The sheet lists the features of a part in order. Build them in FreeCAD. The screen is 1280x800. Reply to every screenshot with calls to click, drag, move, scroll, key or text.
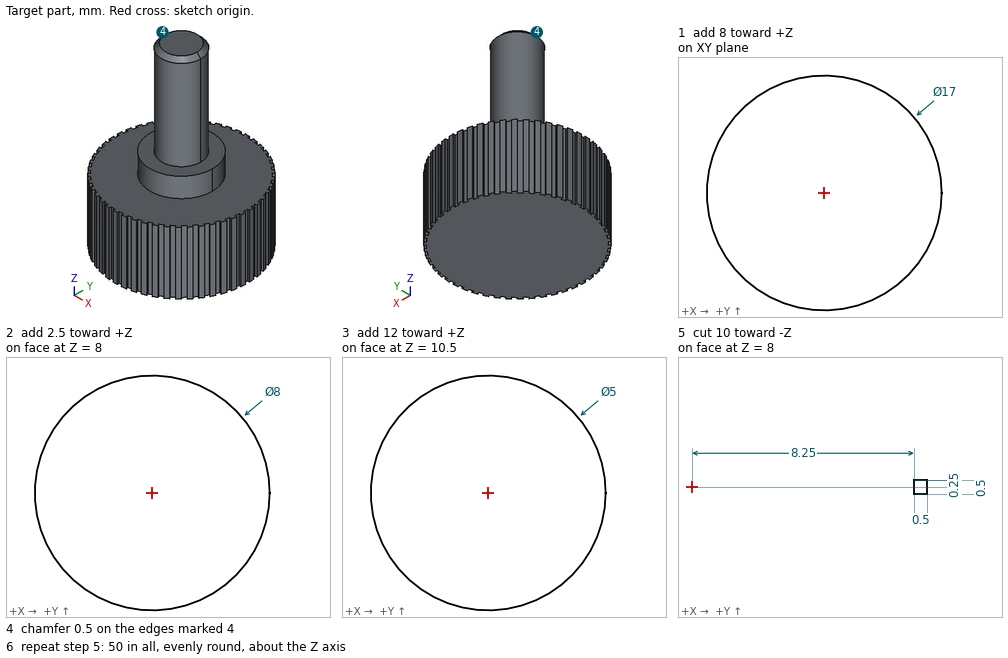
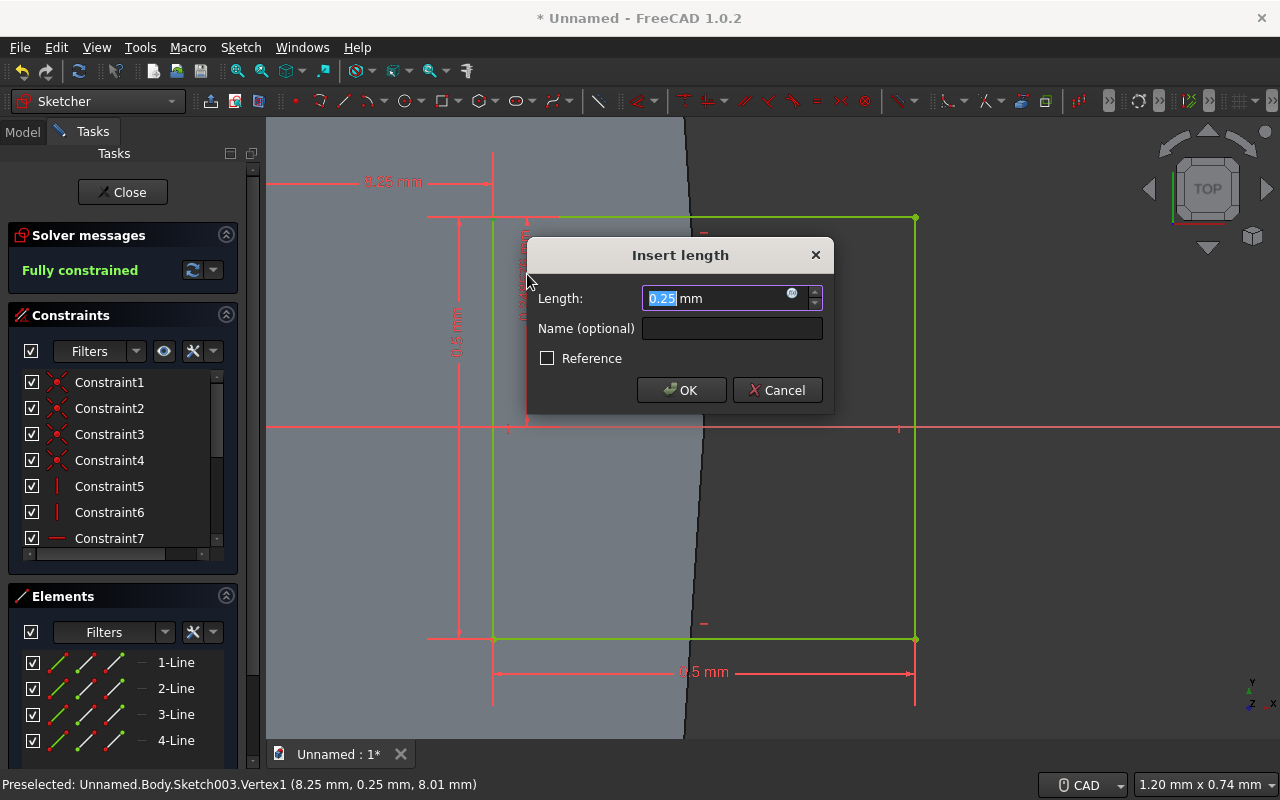
text(0.25)
key(Return)
key(Escape)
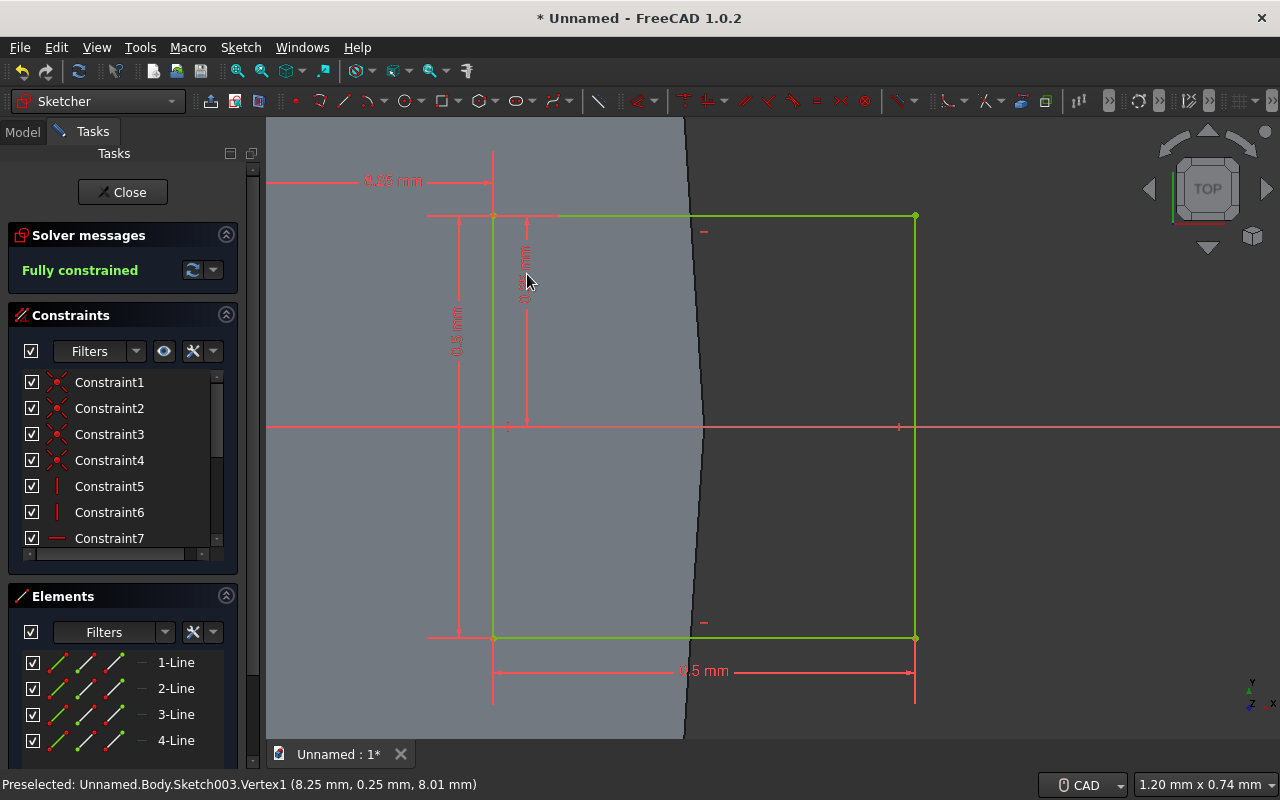
click(123, 192)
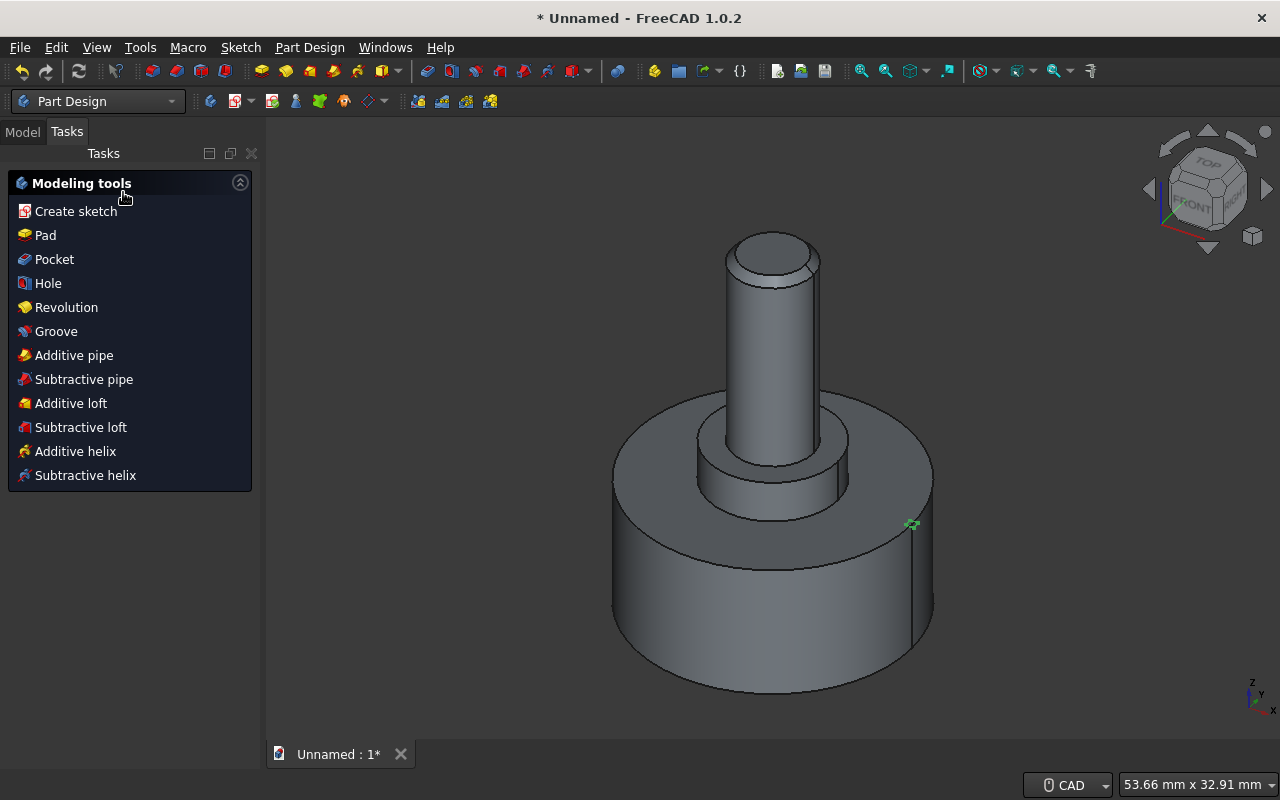
click(428, 72)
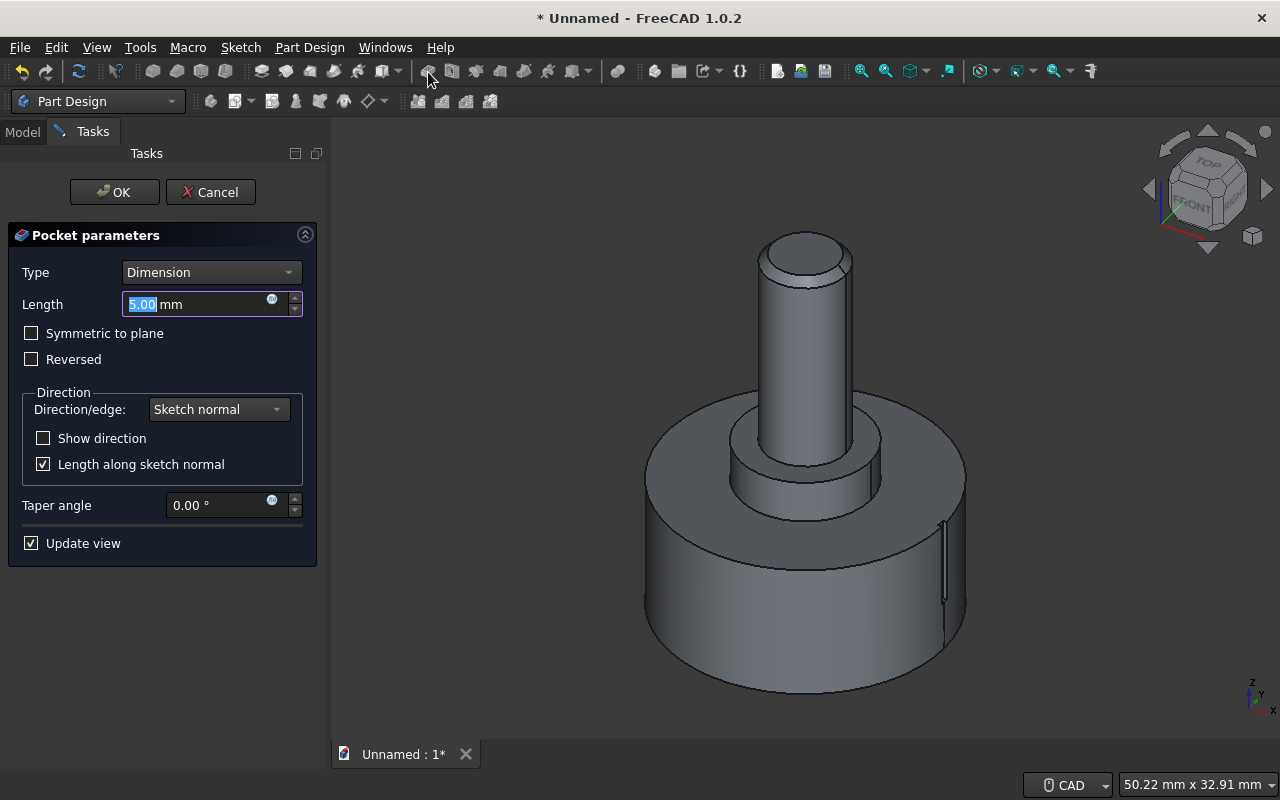
text(10)
key(Tab)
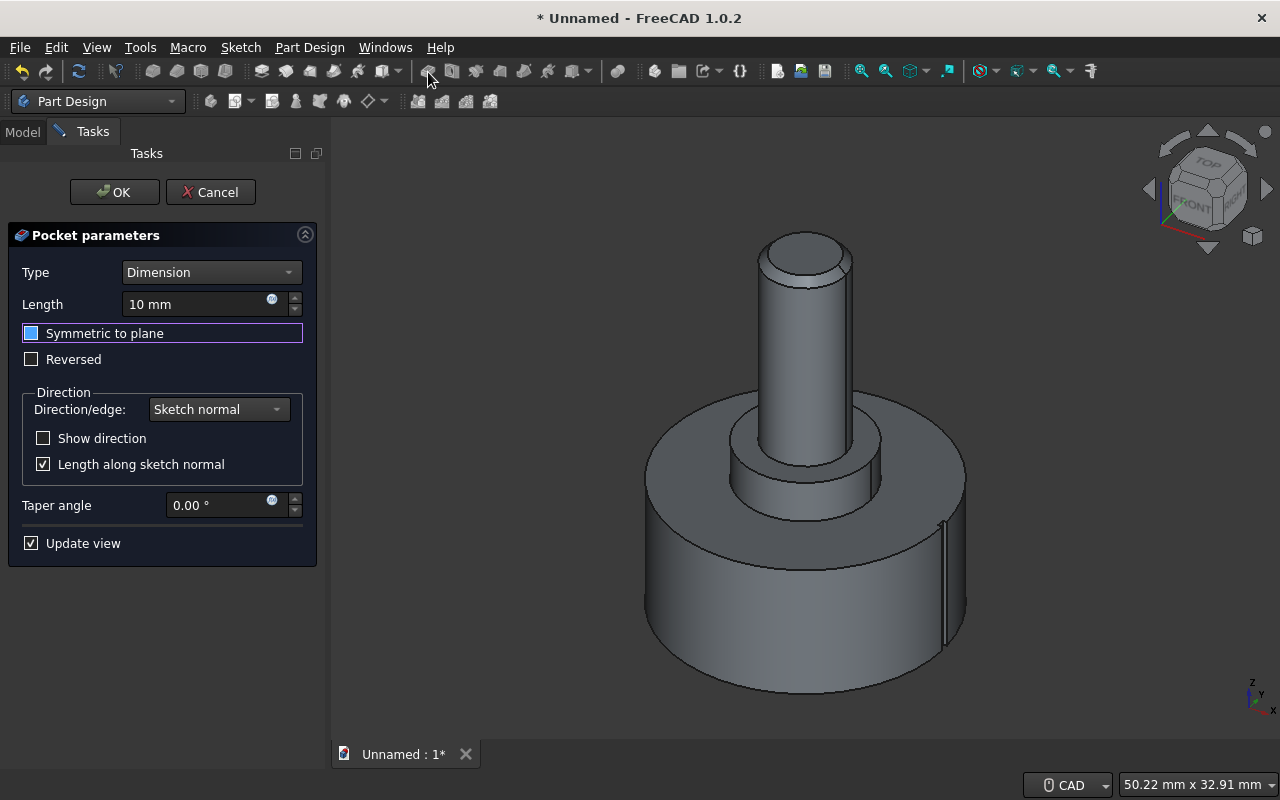
click(115, 192)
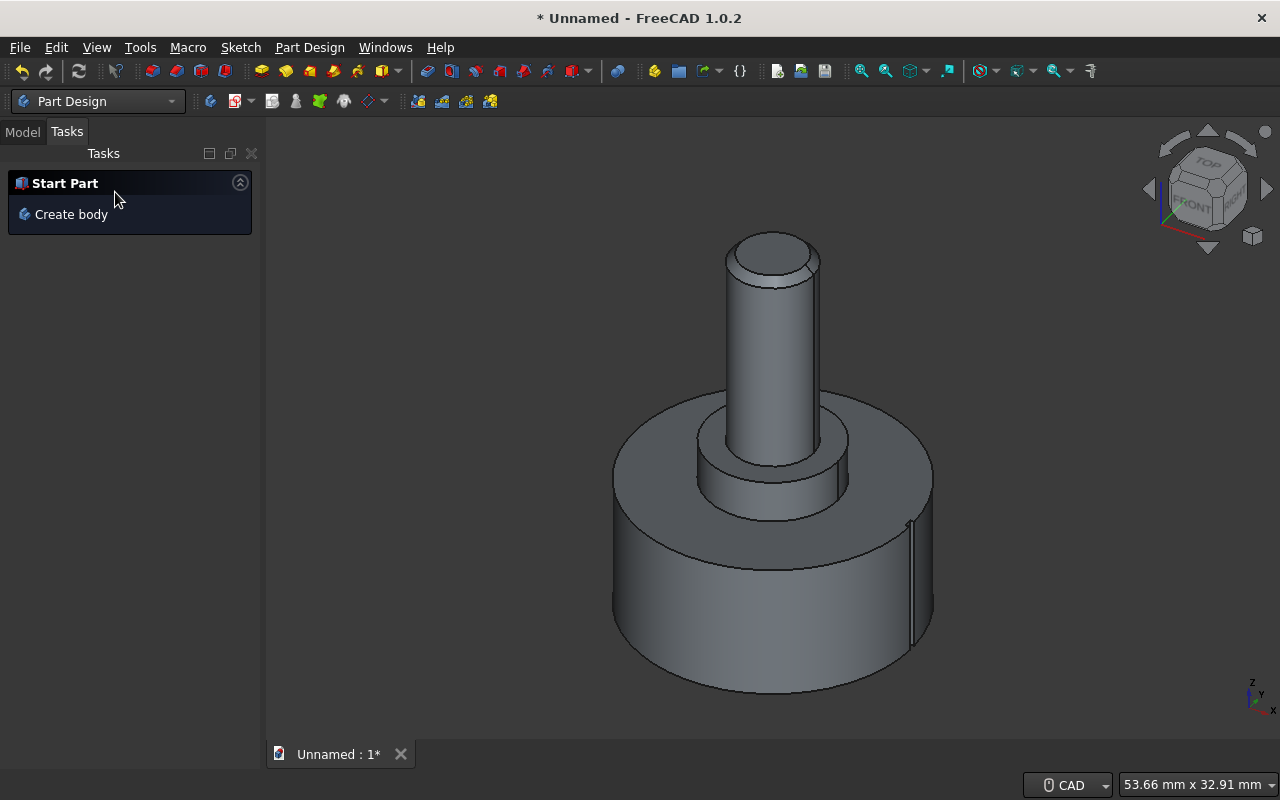
click(23, 131)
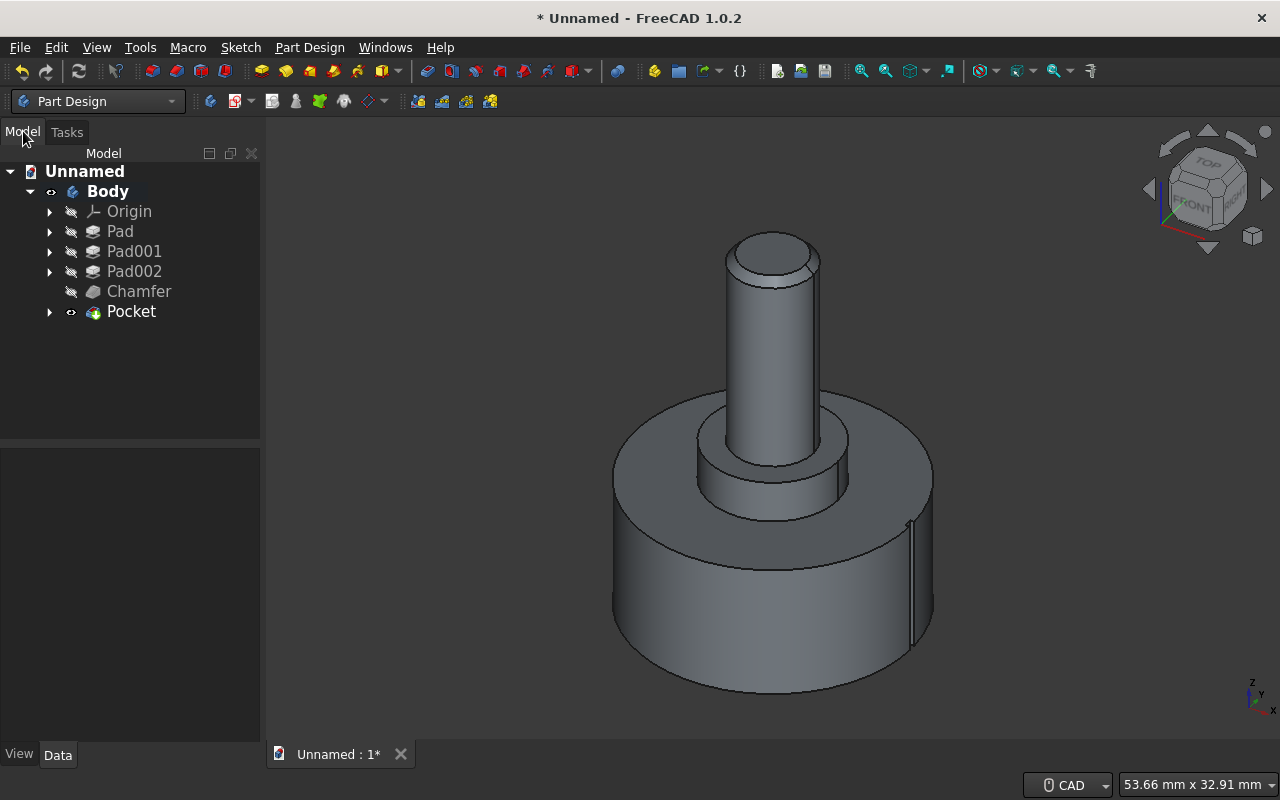
click(116, 312)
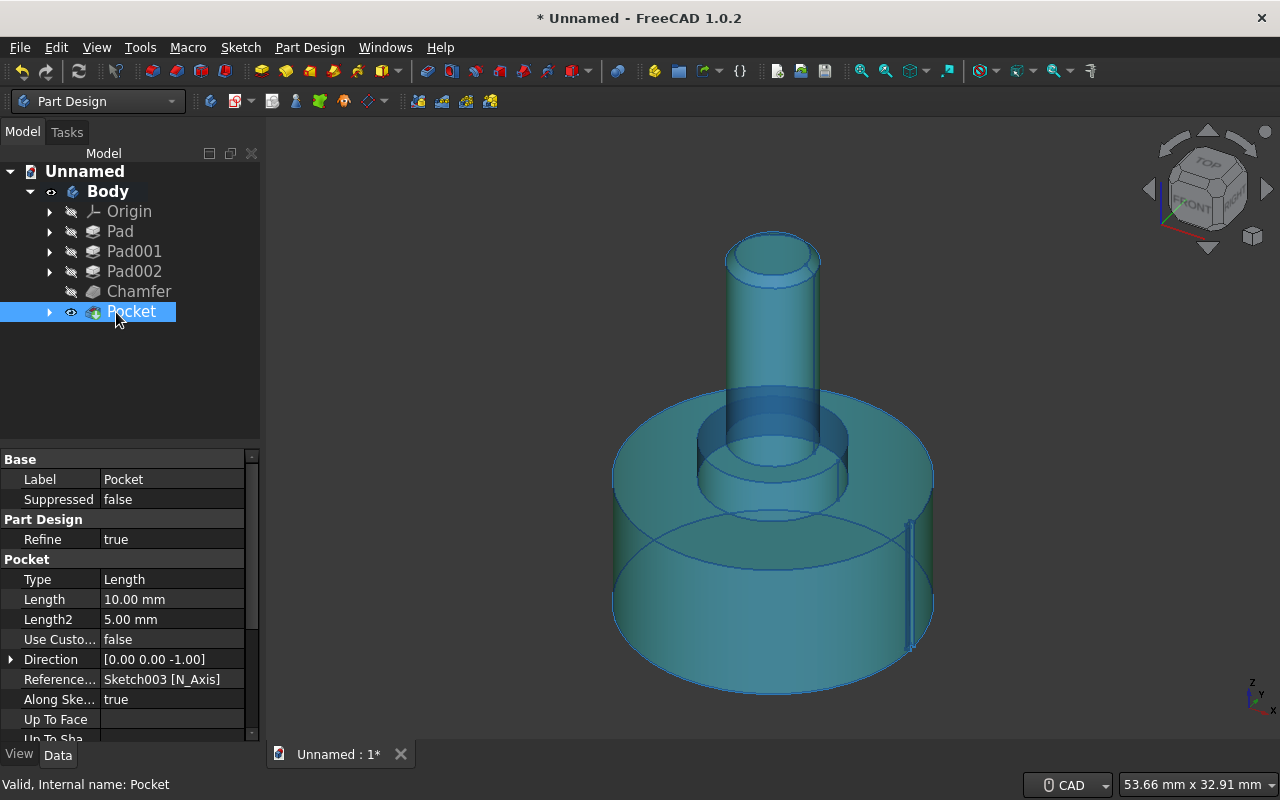
click(466, 102)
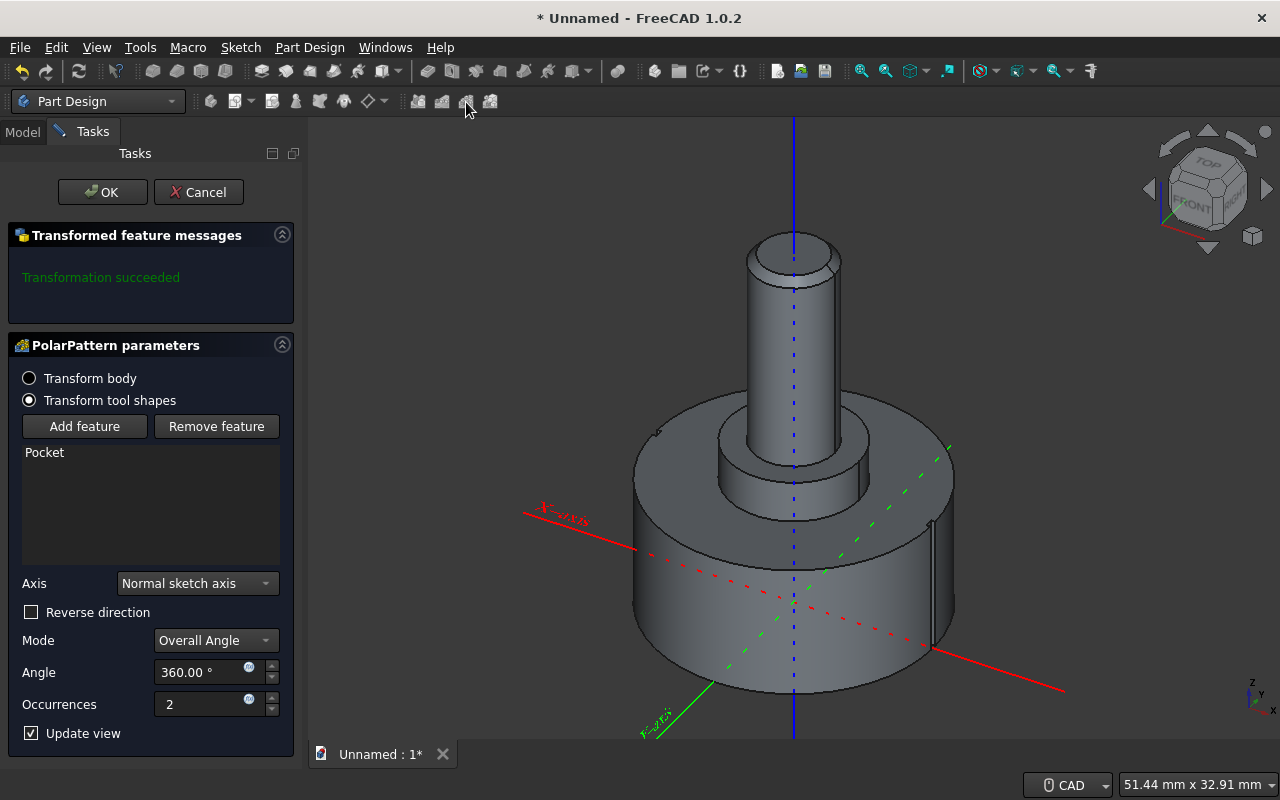
click(198, 584)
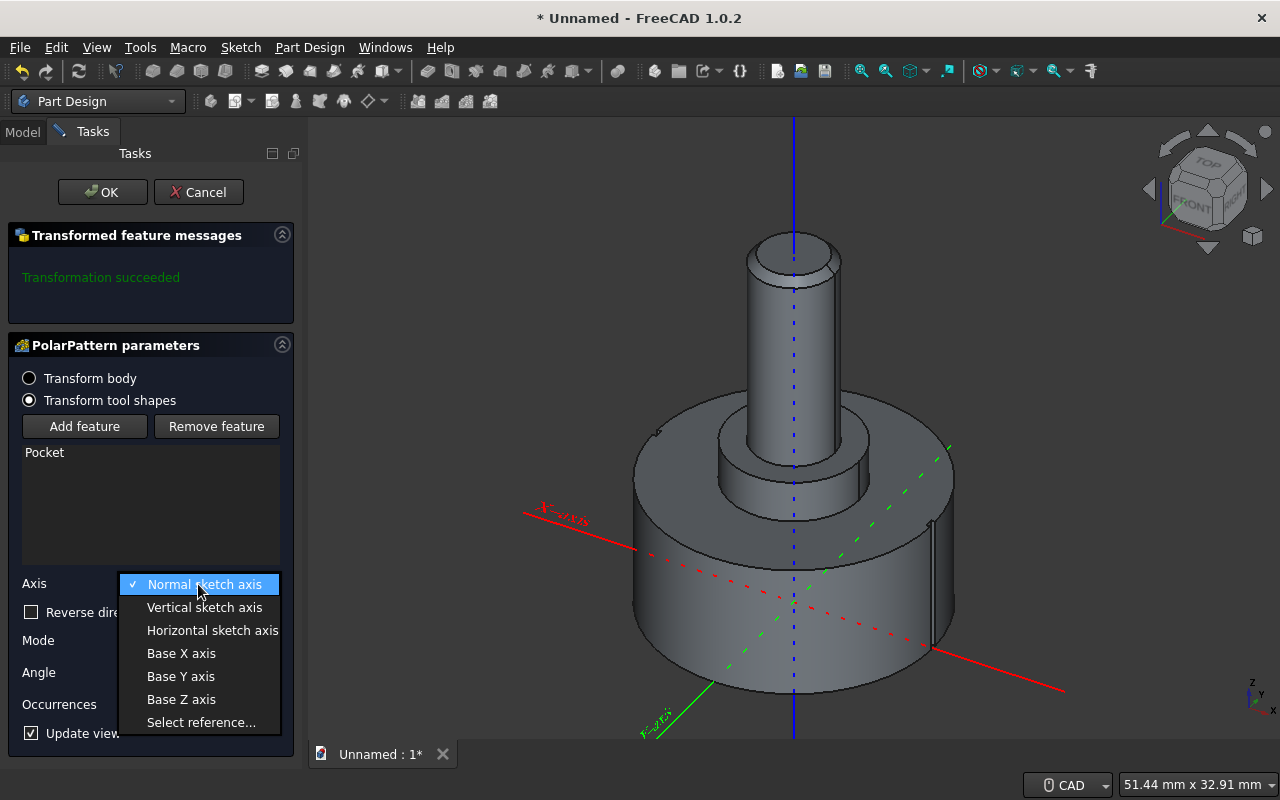
click(198, 700)